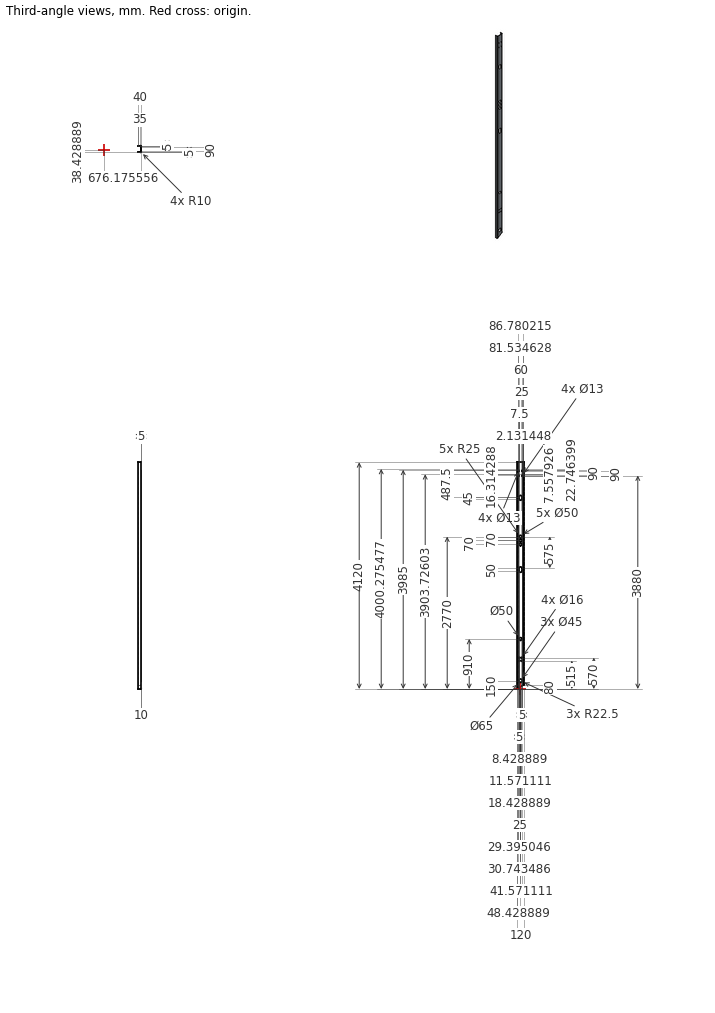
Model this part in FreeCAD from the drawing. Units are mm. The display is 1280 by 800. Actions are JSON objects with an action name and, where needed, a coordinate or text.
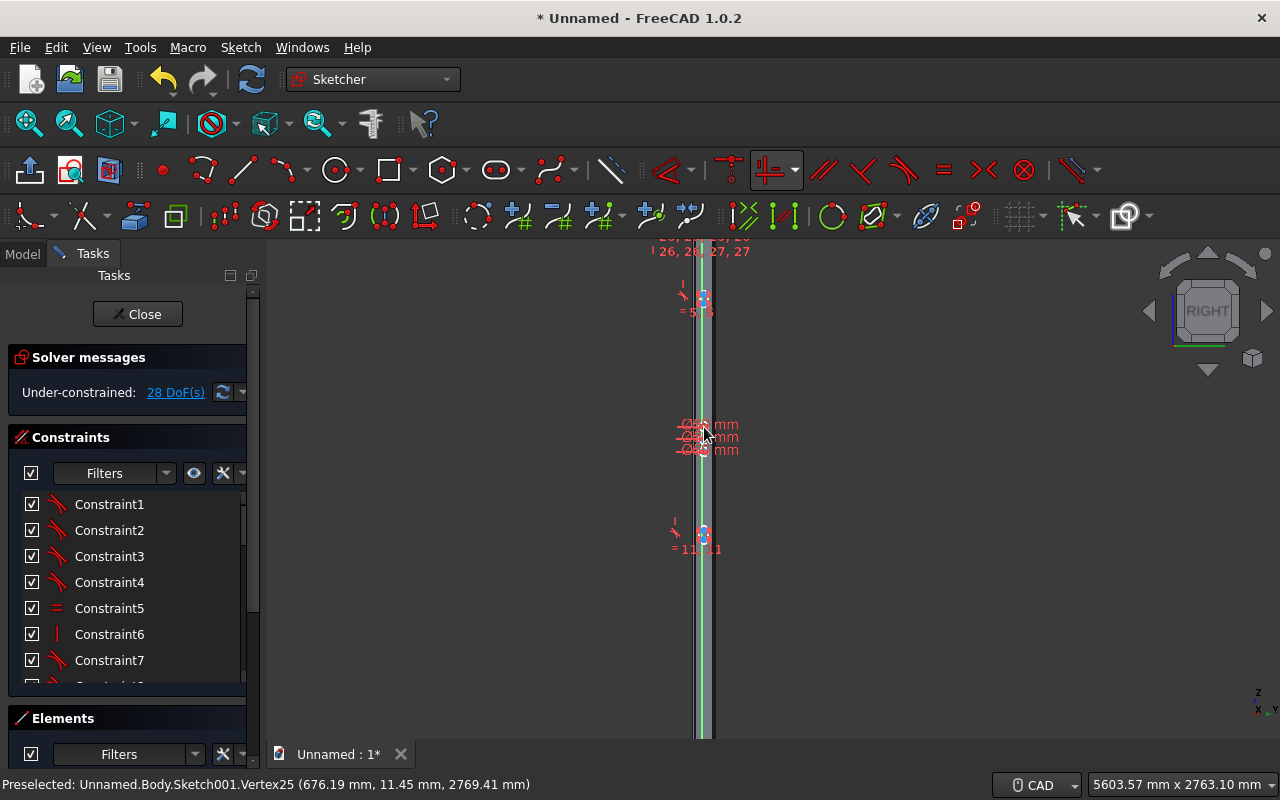
{"action": "left_click", "coordinate": [704, 439]}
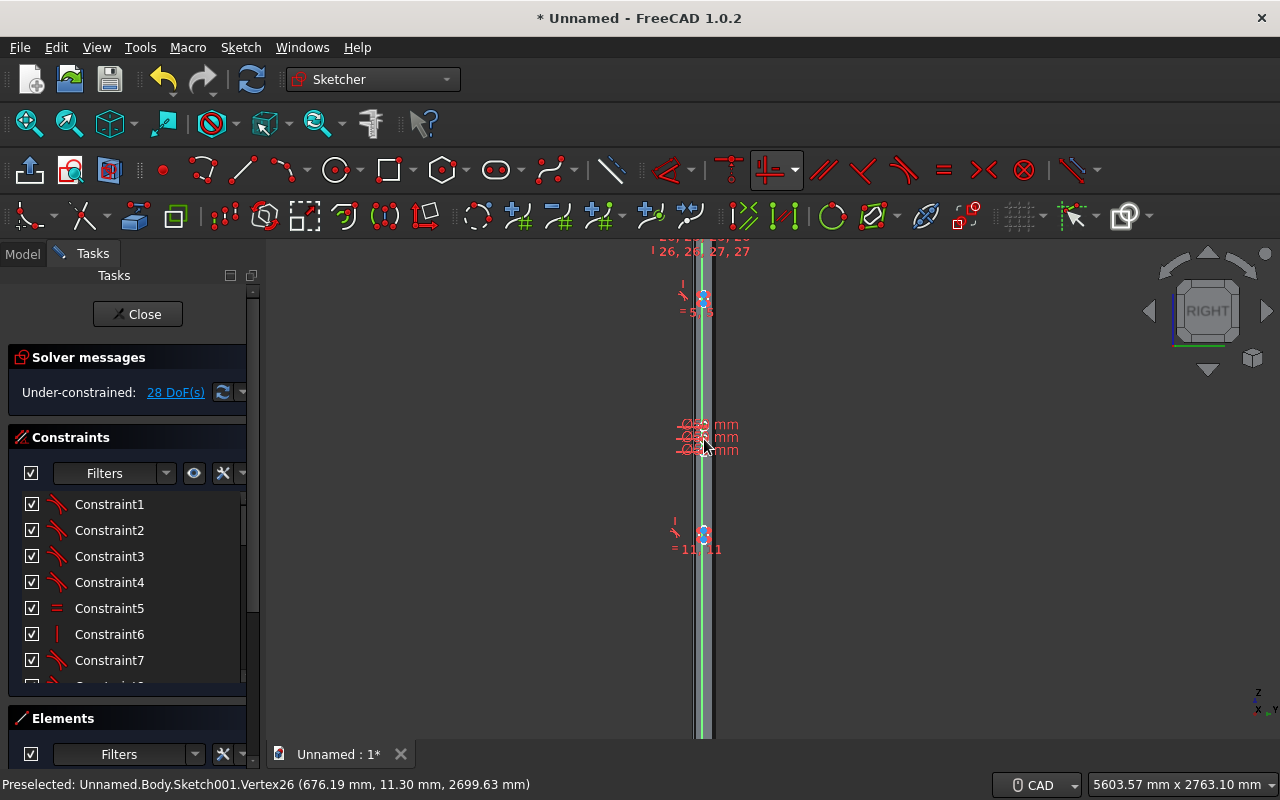
{"action": "key", "text": "v"}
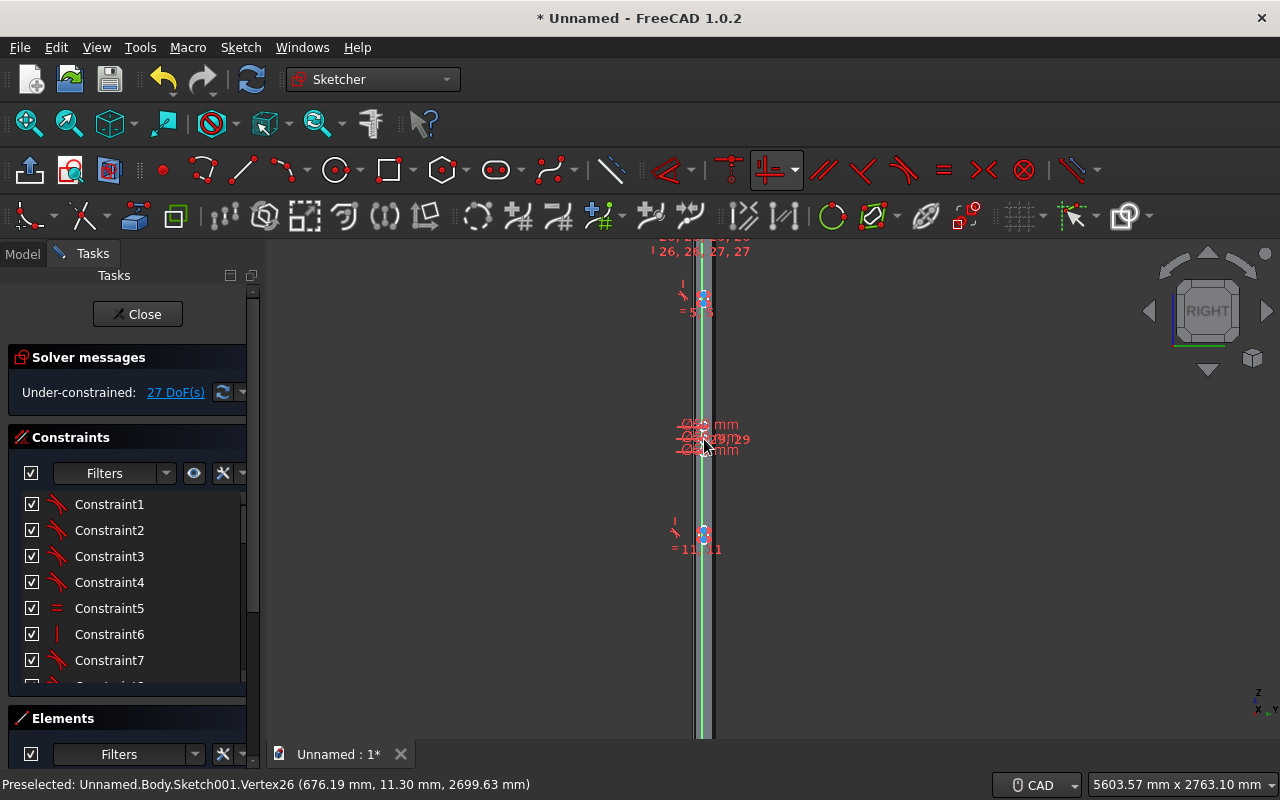
{"action": "scroll", "coordinate": [704, 439], "scroll_direction": "up", "scroll_amount": 4}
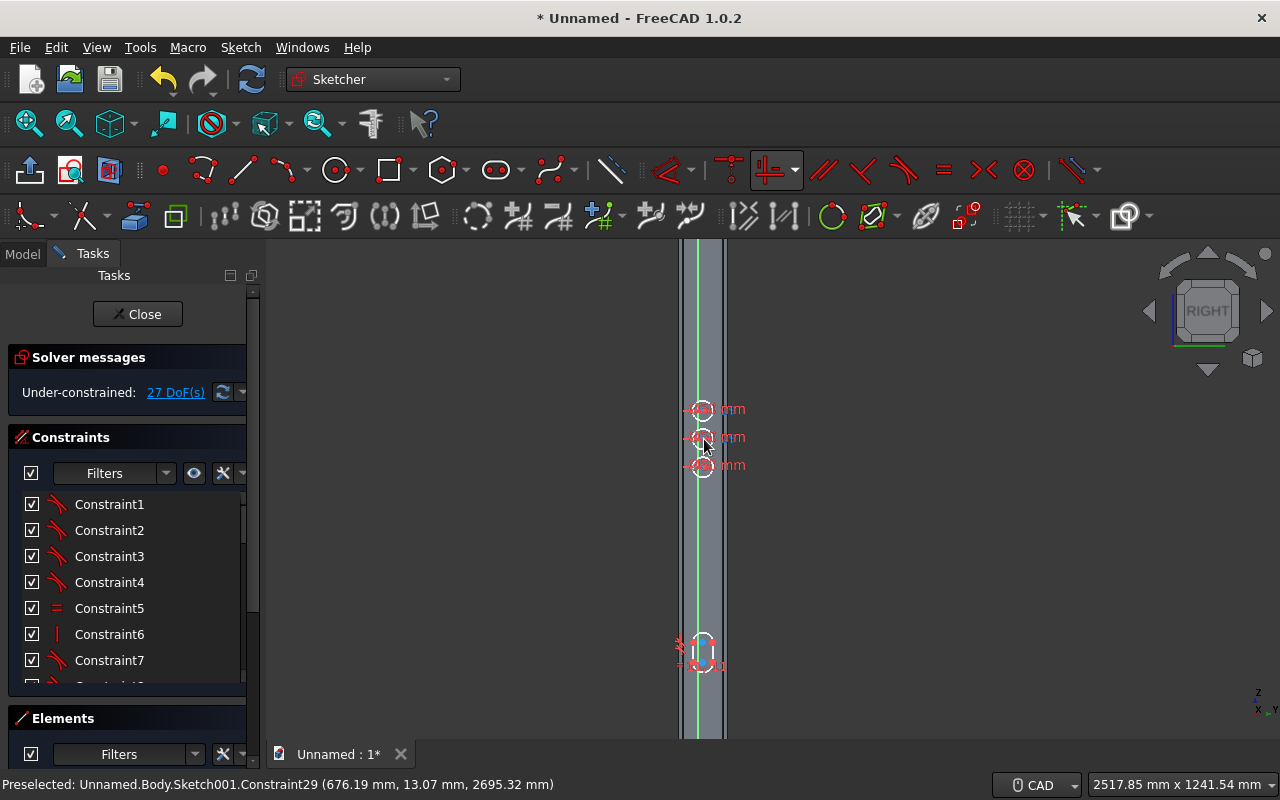
{"action": "left_click", "coordinate": [703, 439]}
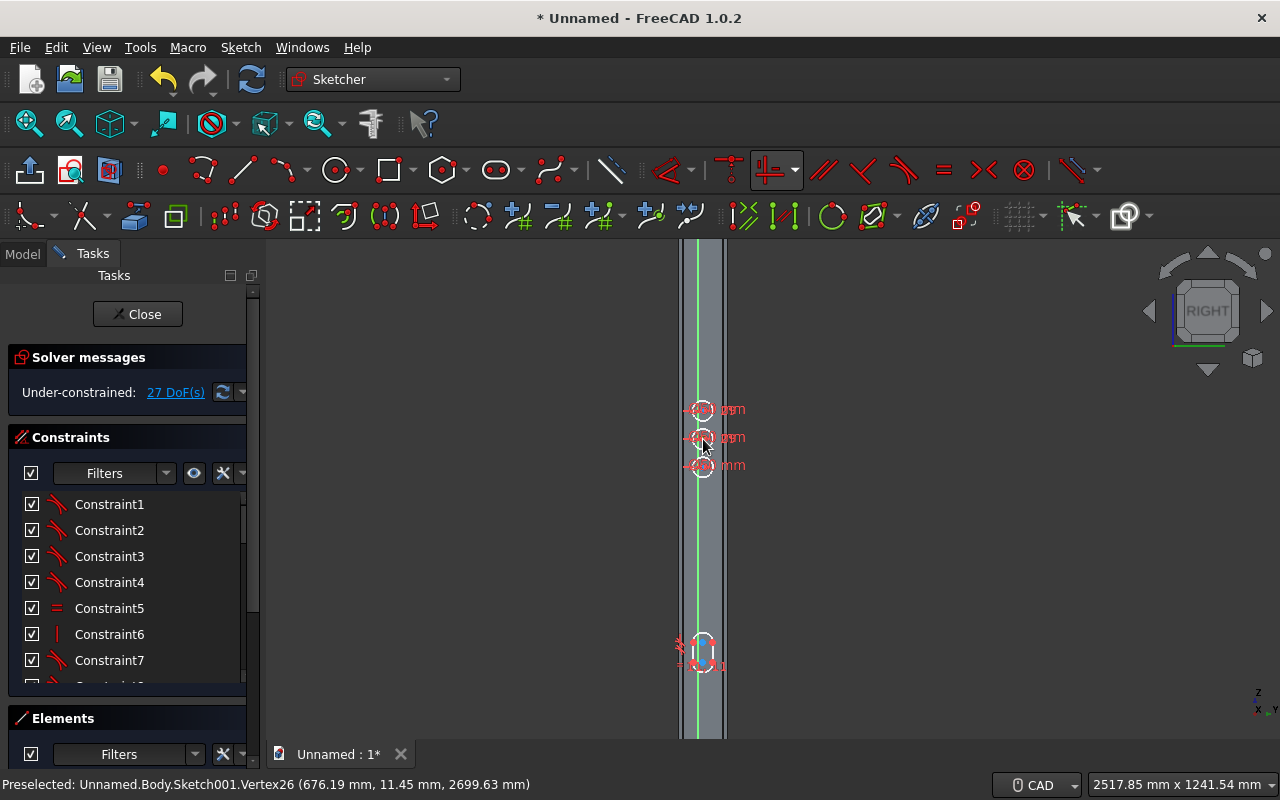
{"action": "left_click", "coordinate": [703, 467]}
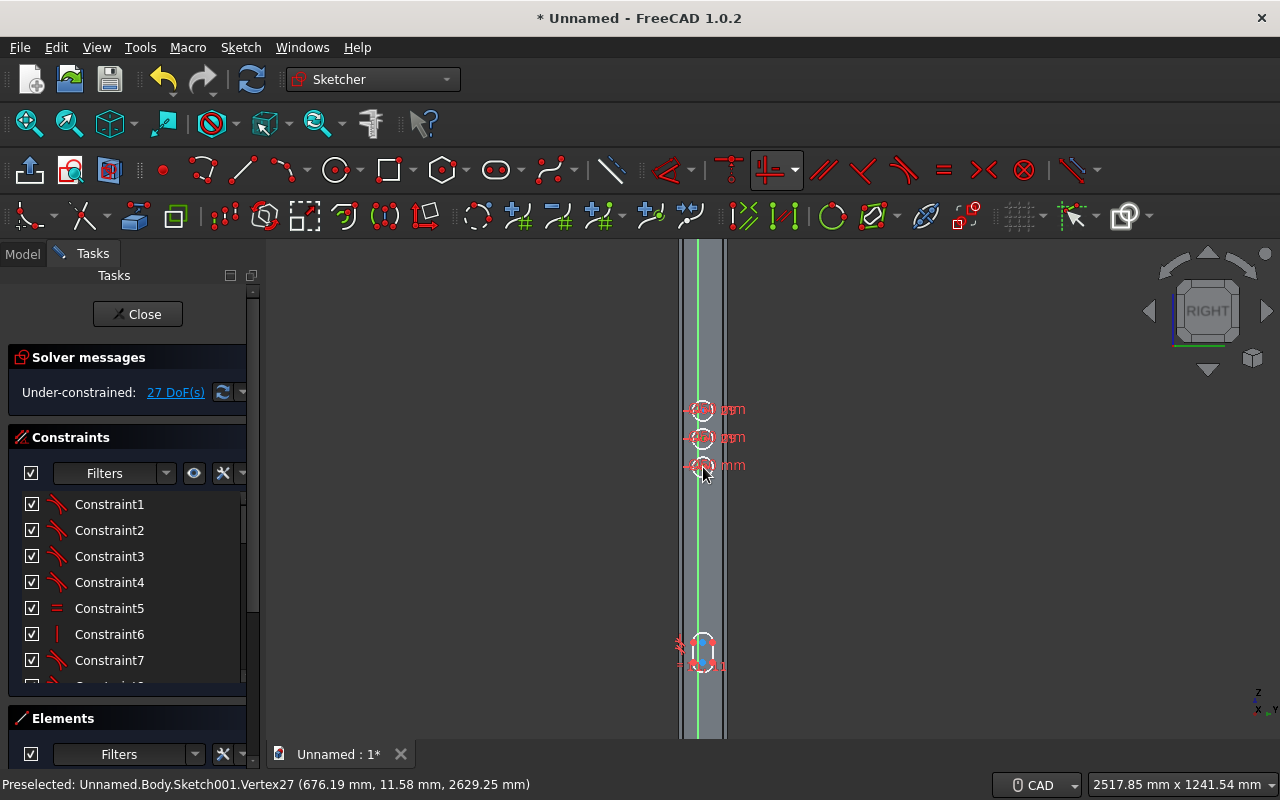
{"action": "key", "text": "v"}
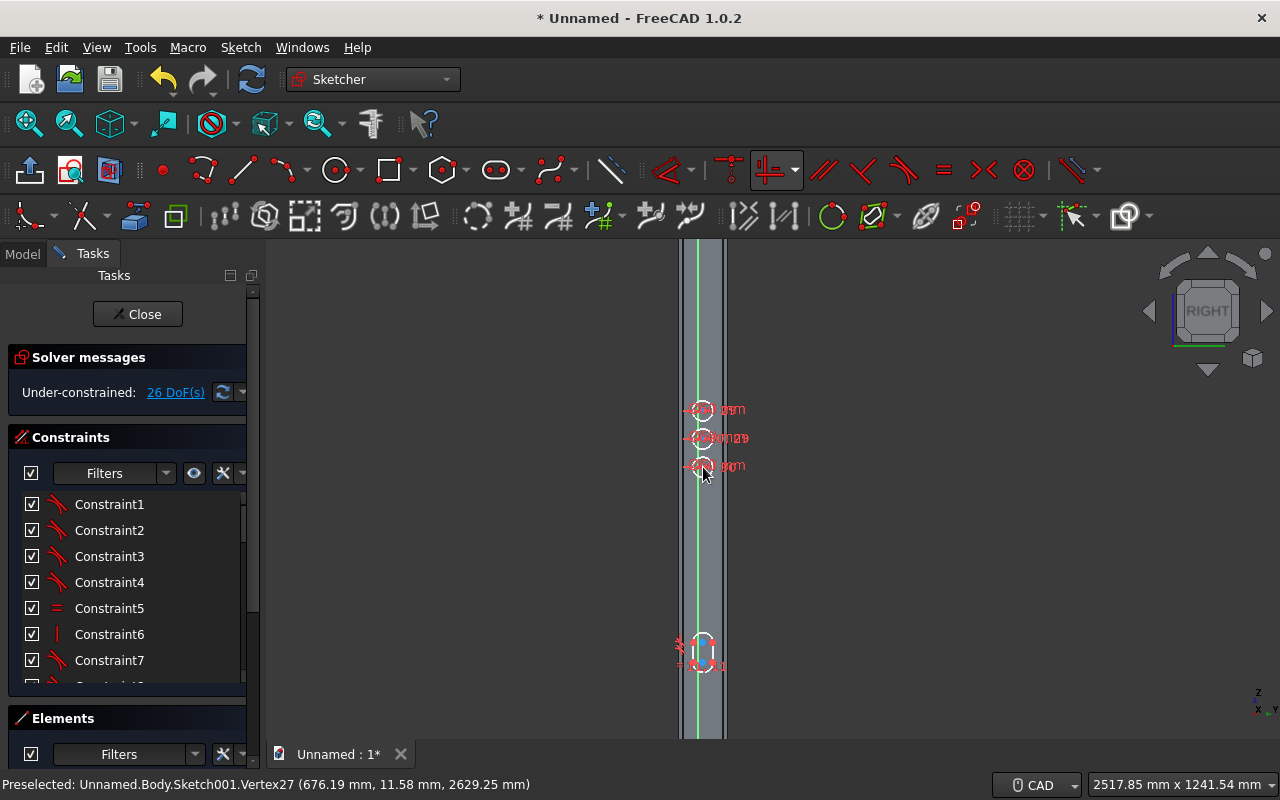
{"action": "scroll", "coordinate": [705, 430], "scroll_direction": "down", "scroll_amount": 8}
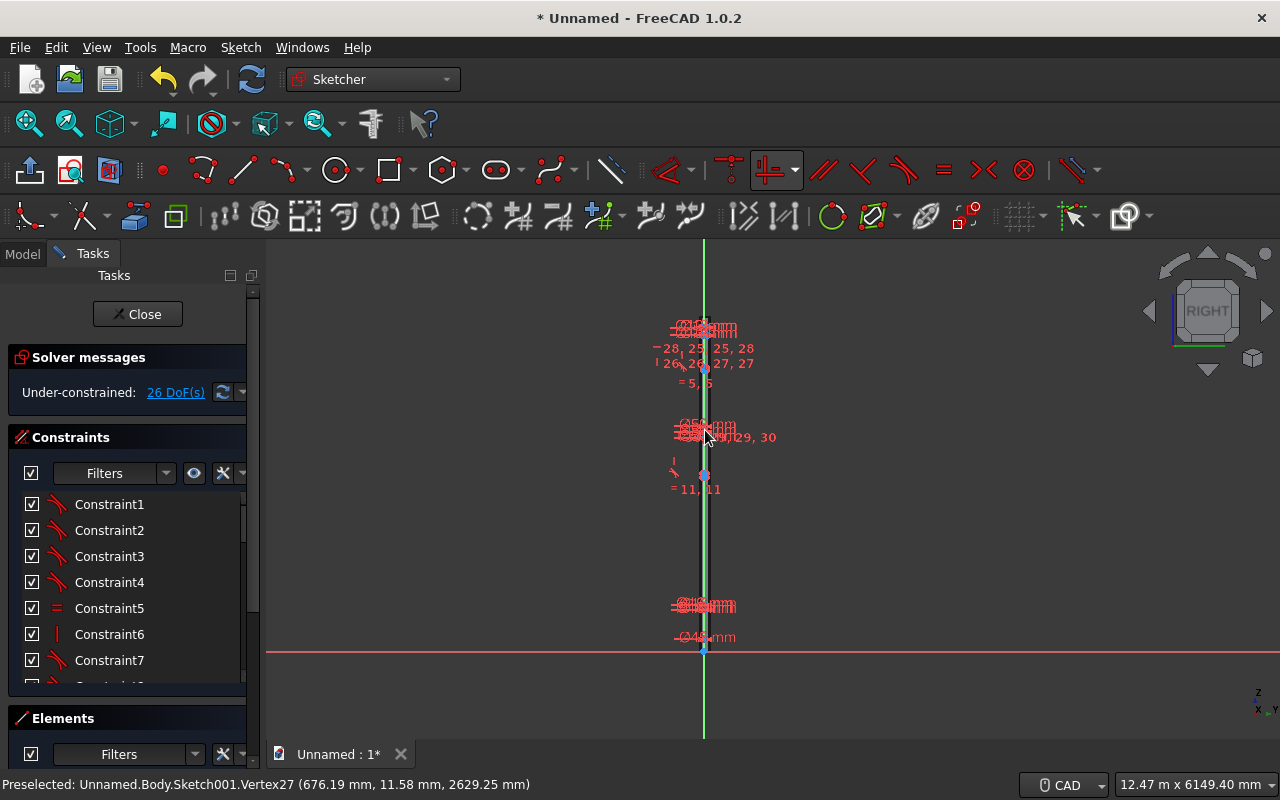
{"action": "scroll", "coordinate": [706, 605], "scroll_direction": "up", "scroll_amount": 7}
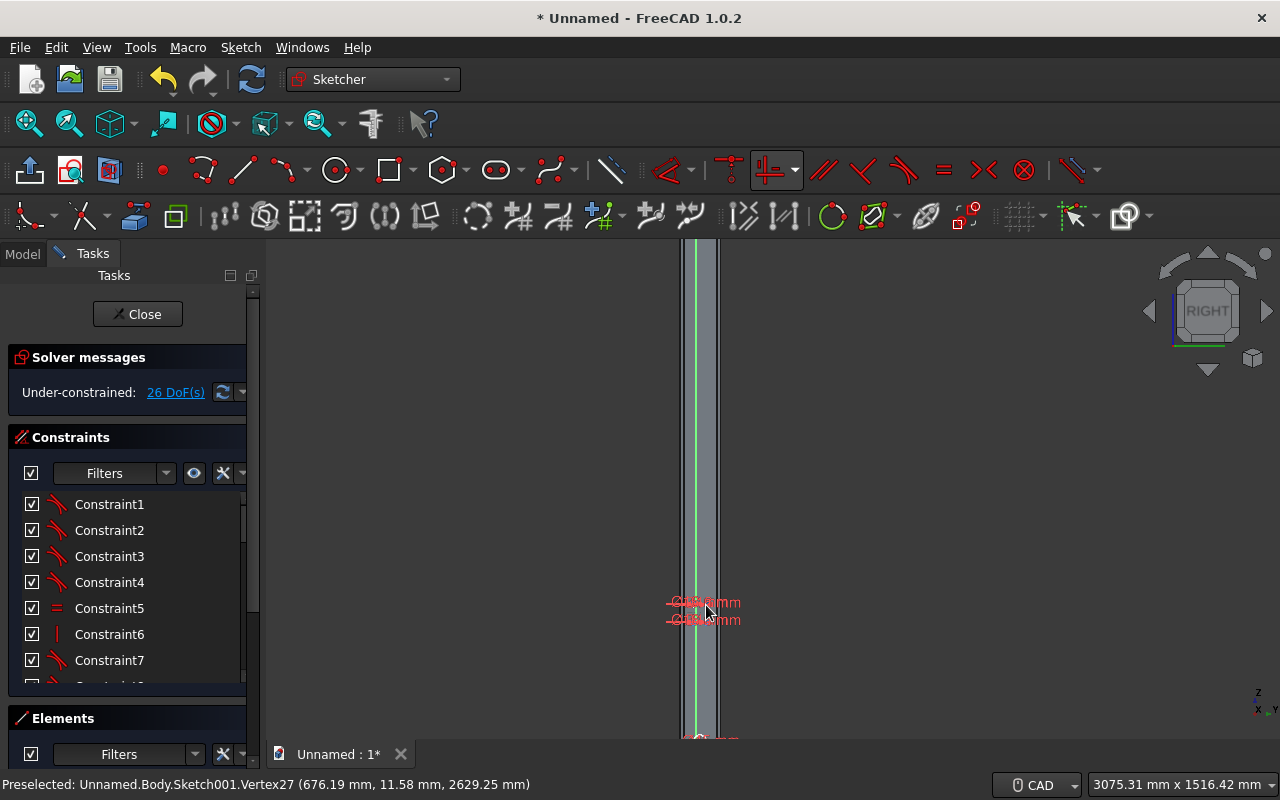
{"action": "left_click", "coordinate": [707, 605]}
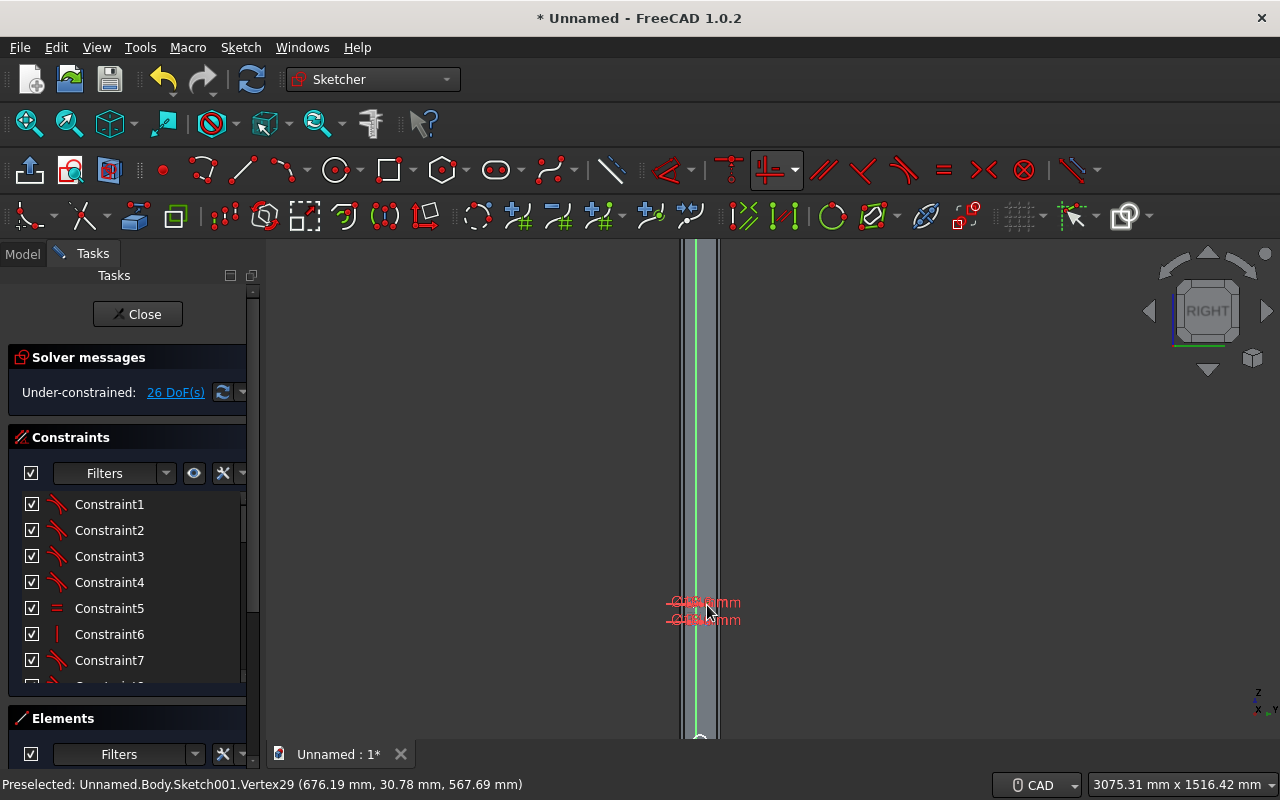
{"action": "left_click", "coordinate": [707, 622]}